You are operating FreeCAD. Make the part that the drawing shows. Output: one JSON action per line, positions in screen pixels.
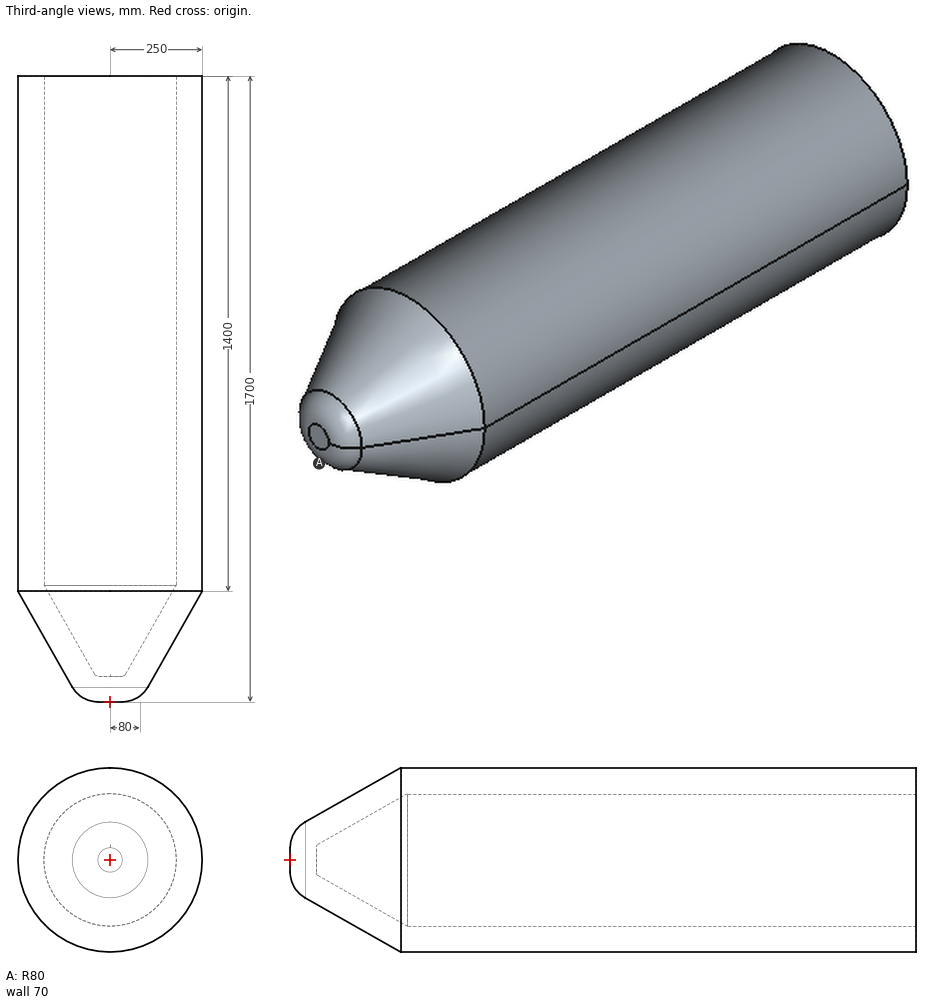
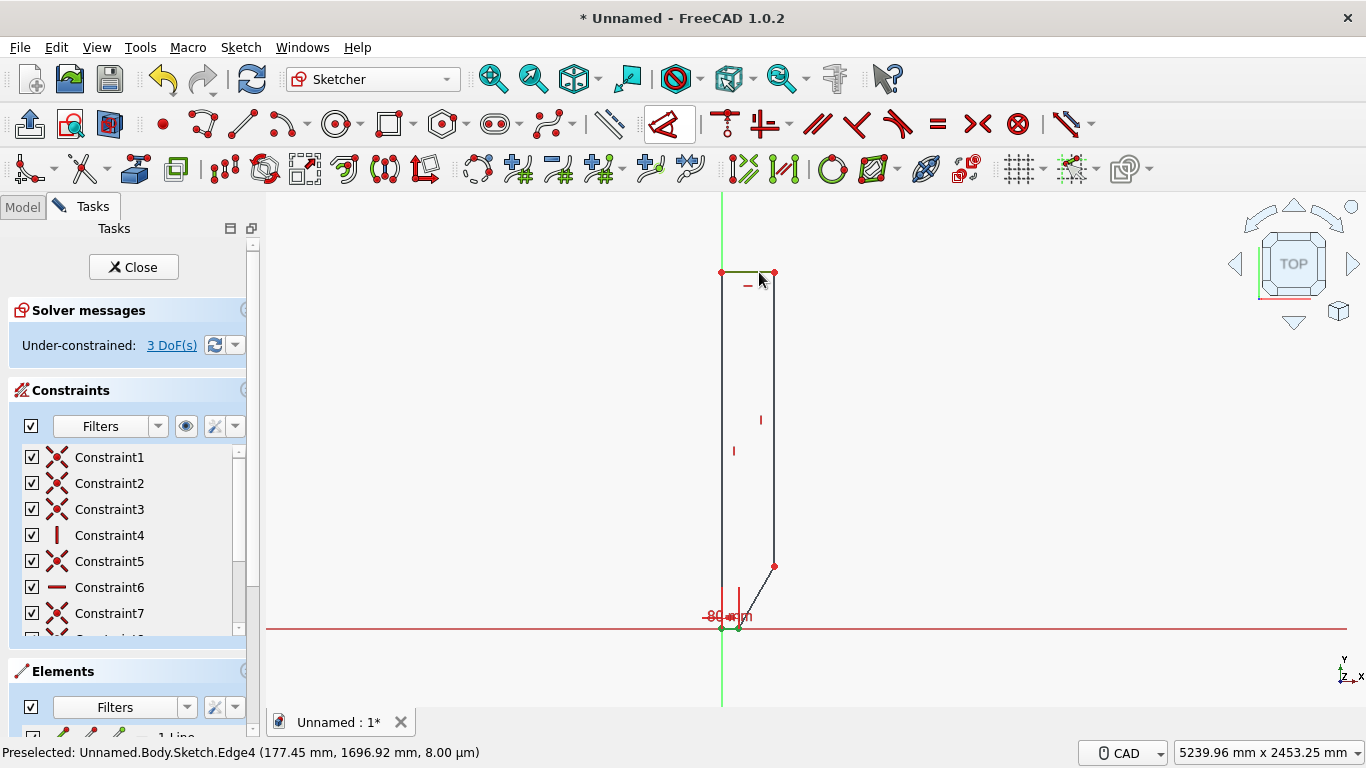
{"action": "key", "text": "l"}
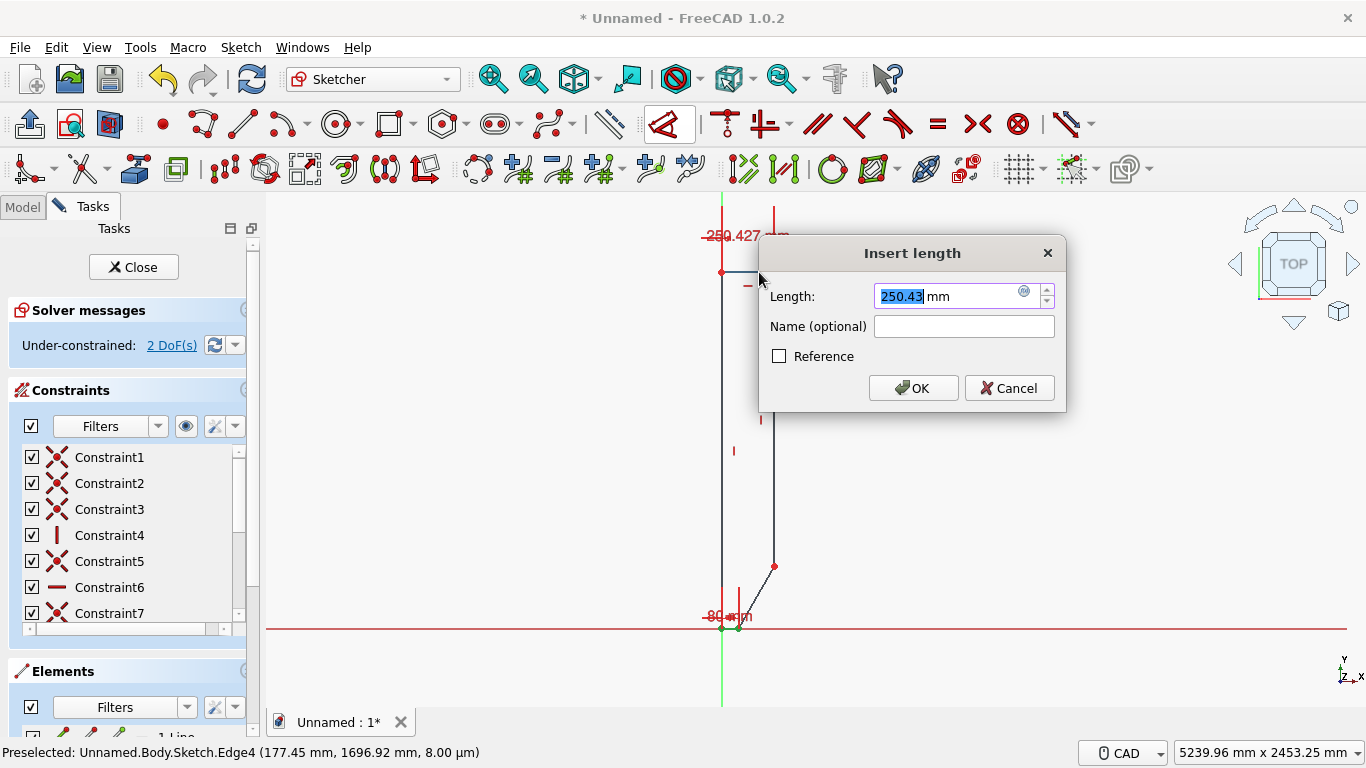
{"action": "type", "text": "250"}
{"action": "key", "text": "Return"}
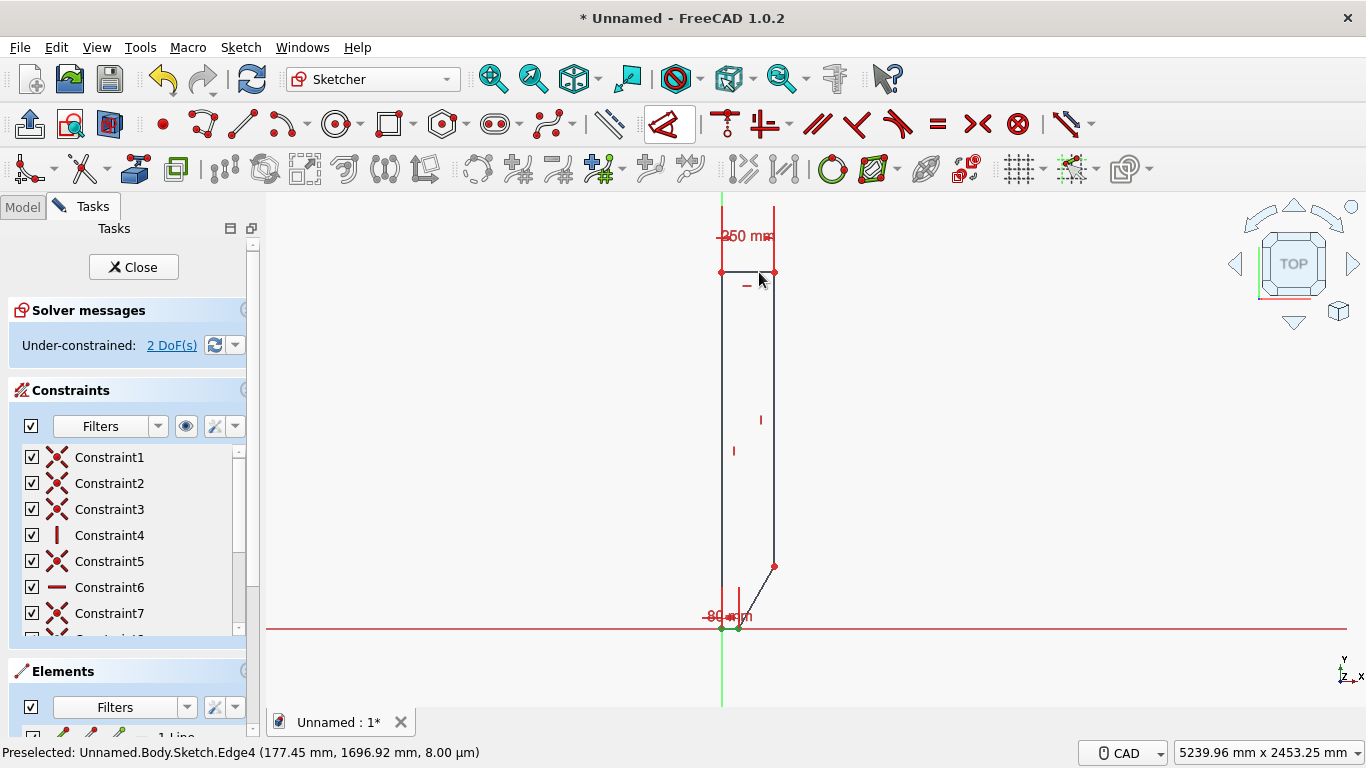
{"action": "left_click", "coordinate": [774, 478]}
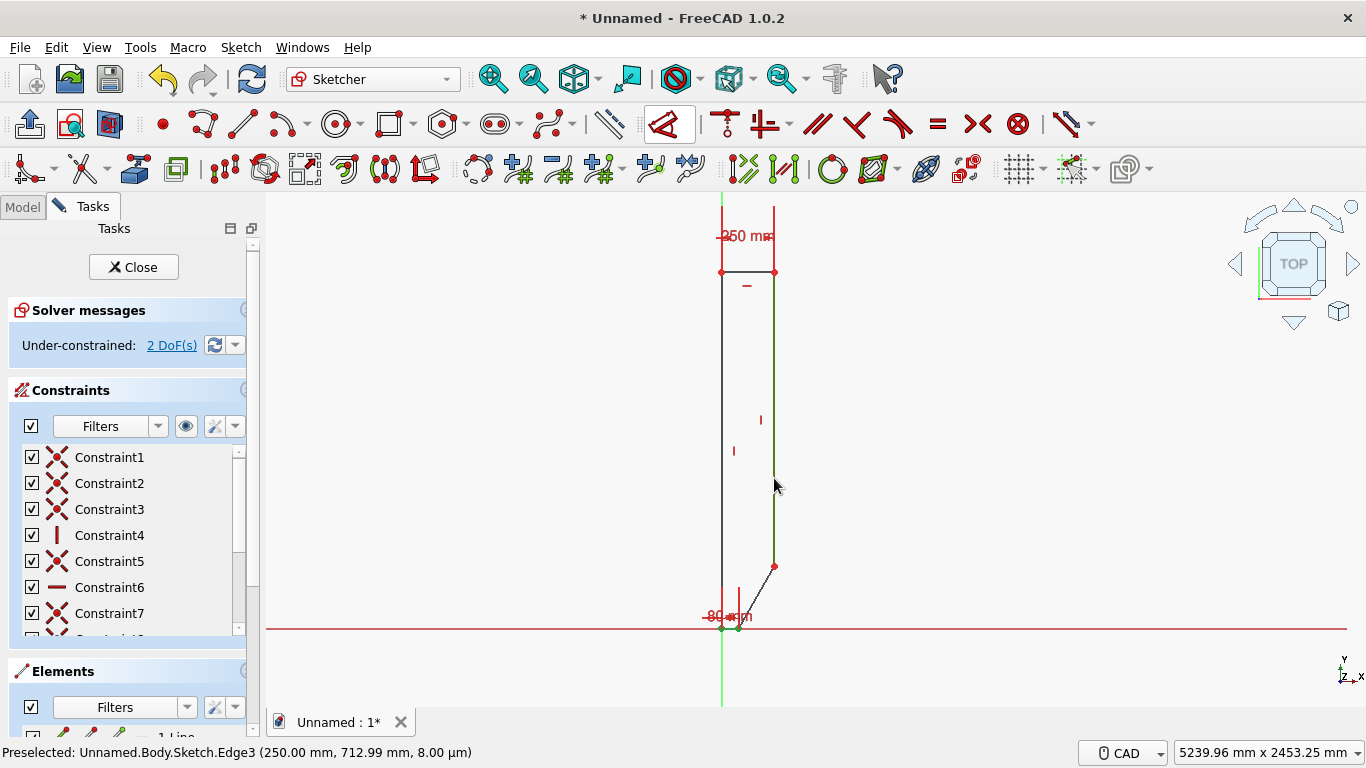
{"action": "key", "text": "i"}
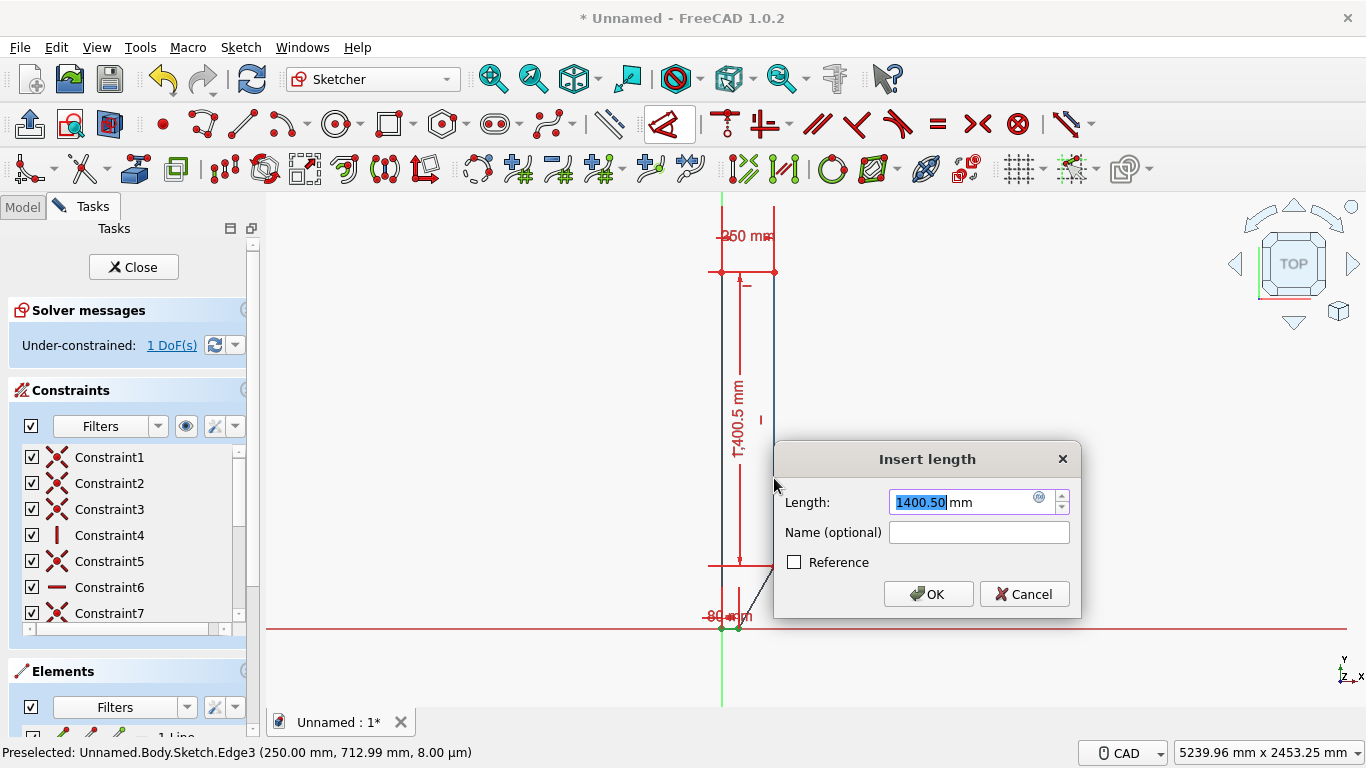
{"action": "type", "text": "1400"}
{"action": "key", "text": "Return"}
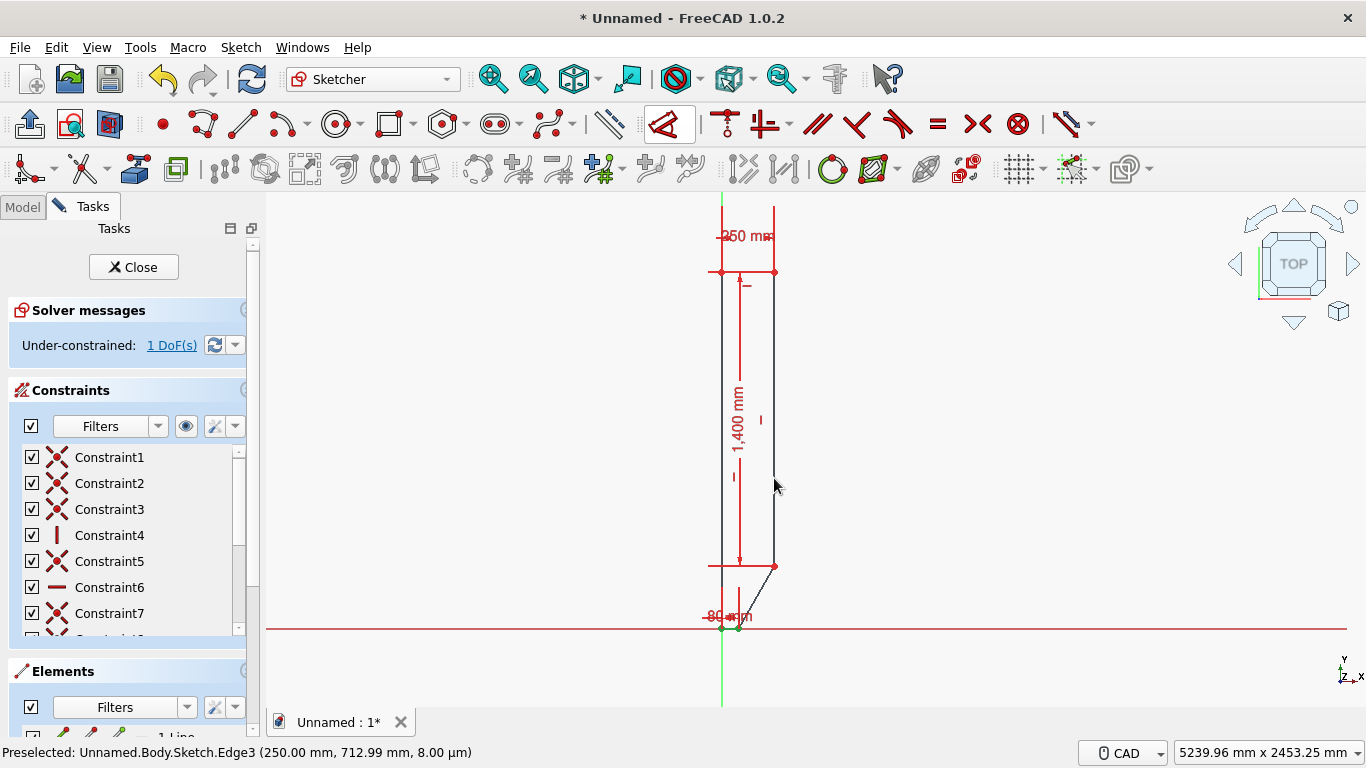
{"action": "left_click", "coordinate": [722, 379]}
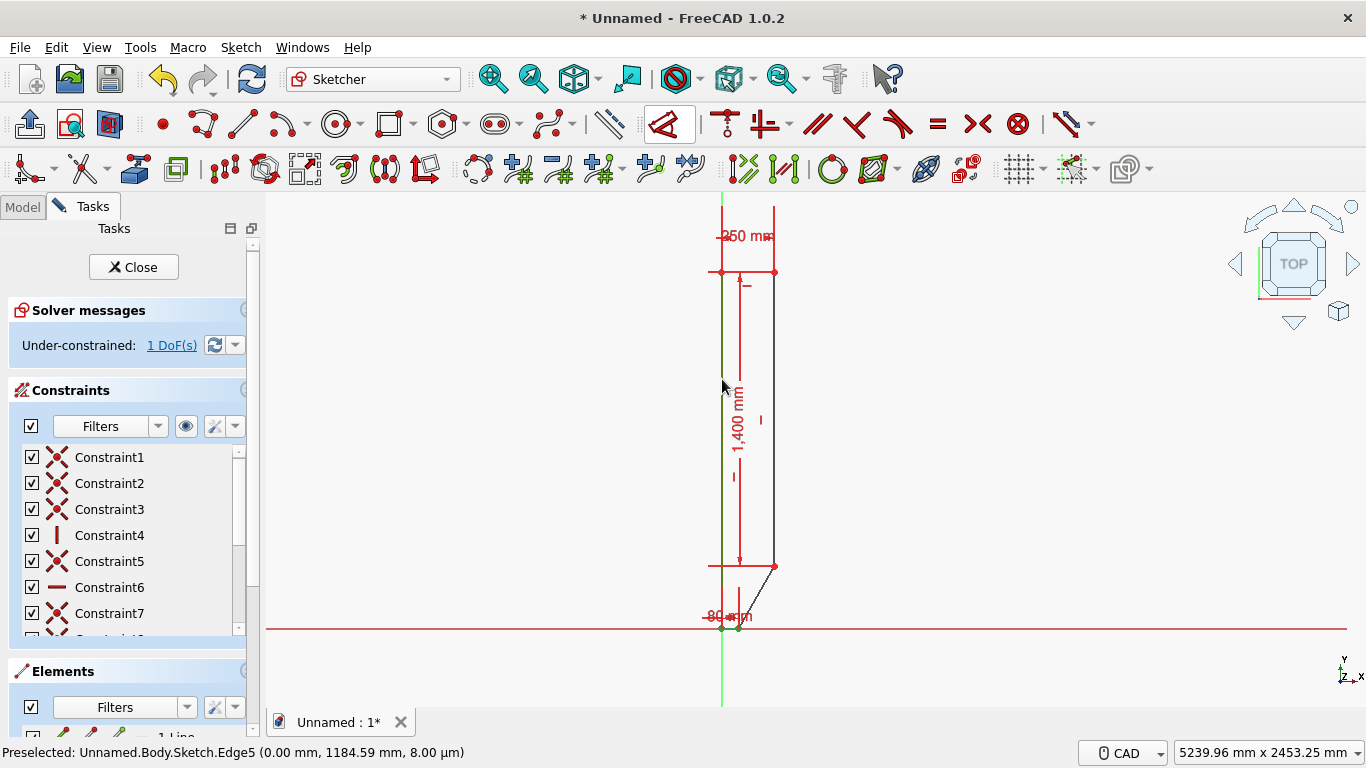
{"action": "left_click", "coordinate": [690, 124]}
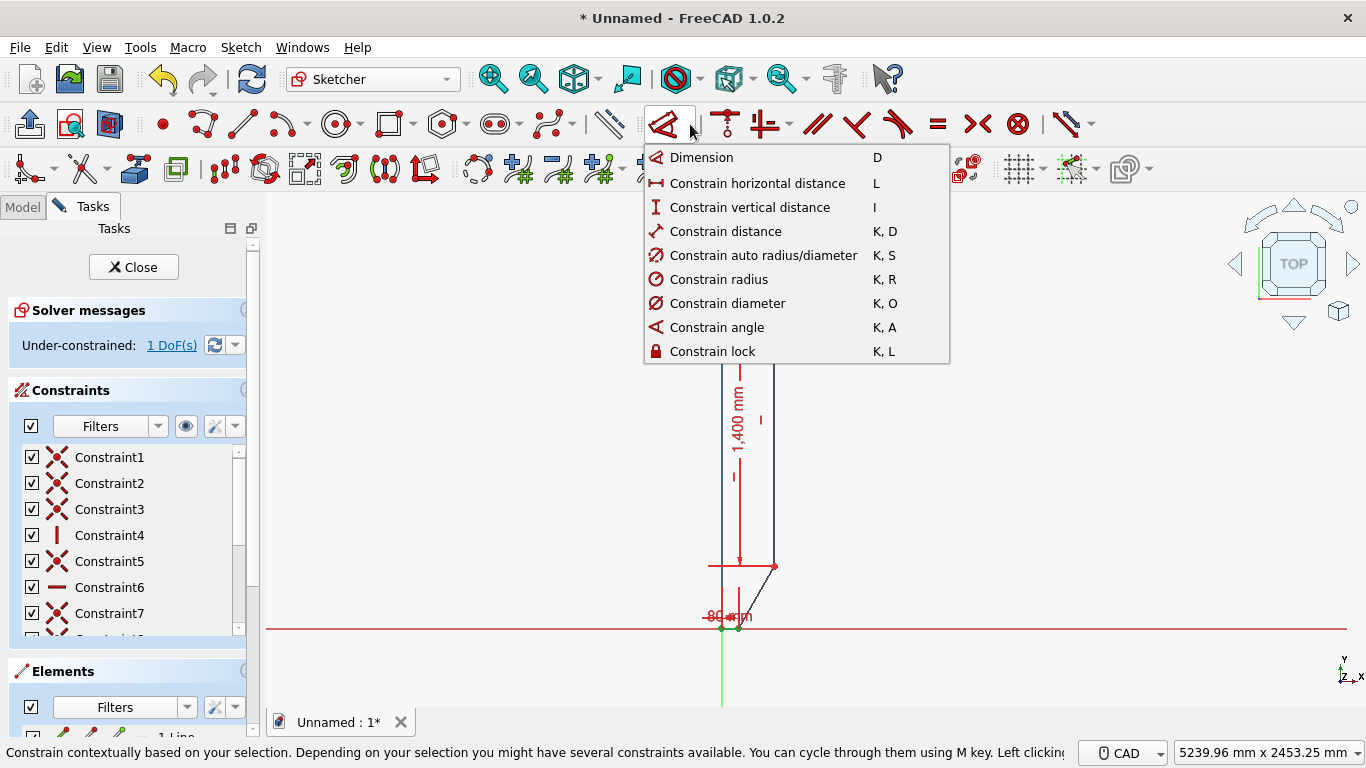
{"action": "left_click", "coordinate": [797, 207]}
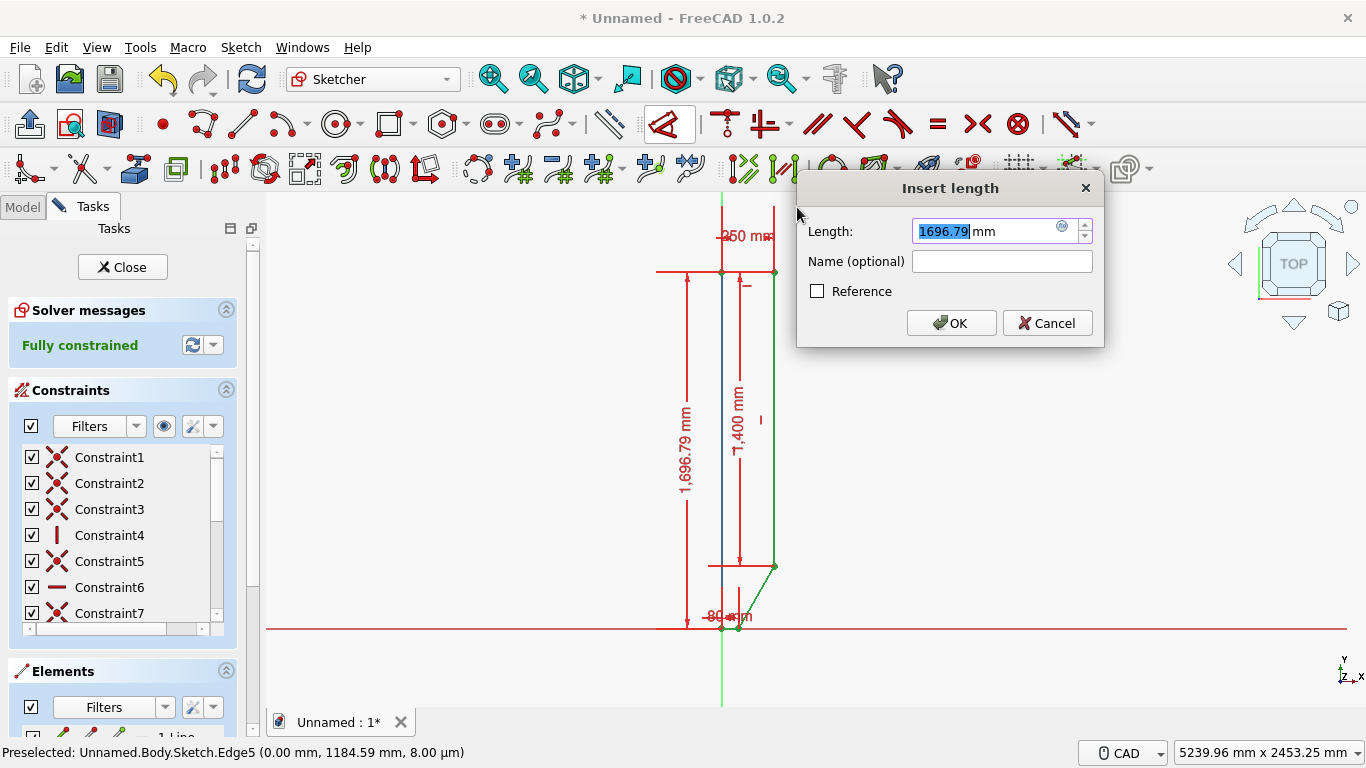
{"action": "type", "text": "1700"}
{"action": "key", "text": "Return"}